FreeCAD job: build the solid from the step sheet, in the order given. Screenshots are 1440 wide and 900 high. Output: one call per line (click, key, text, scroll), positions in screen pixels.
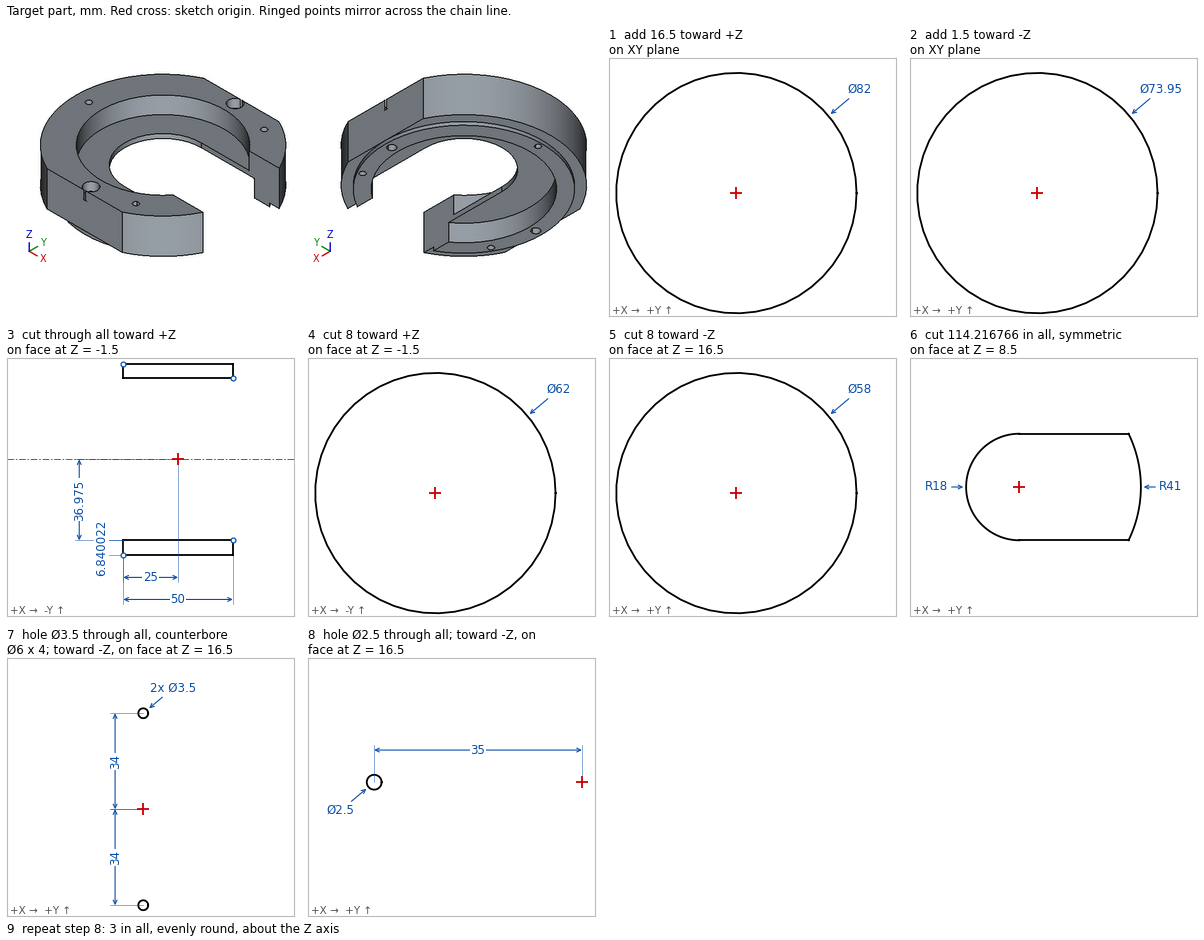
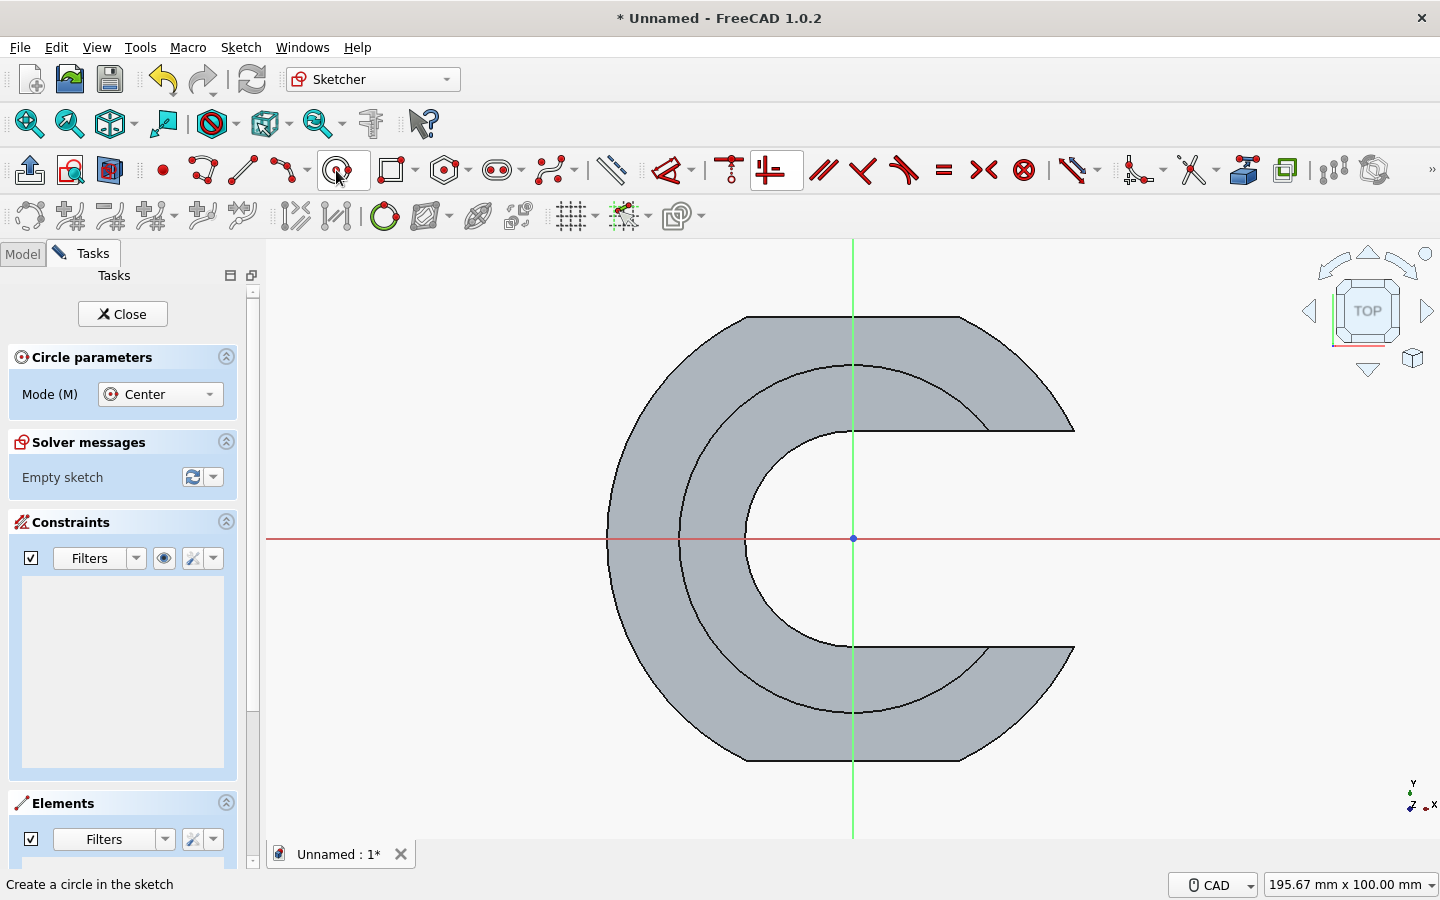
scroll(853, 335, up, 4)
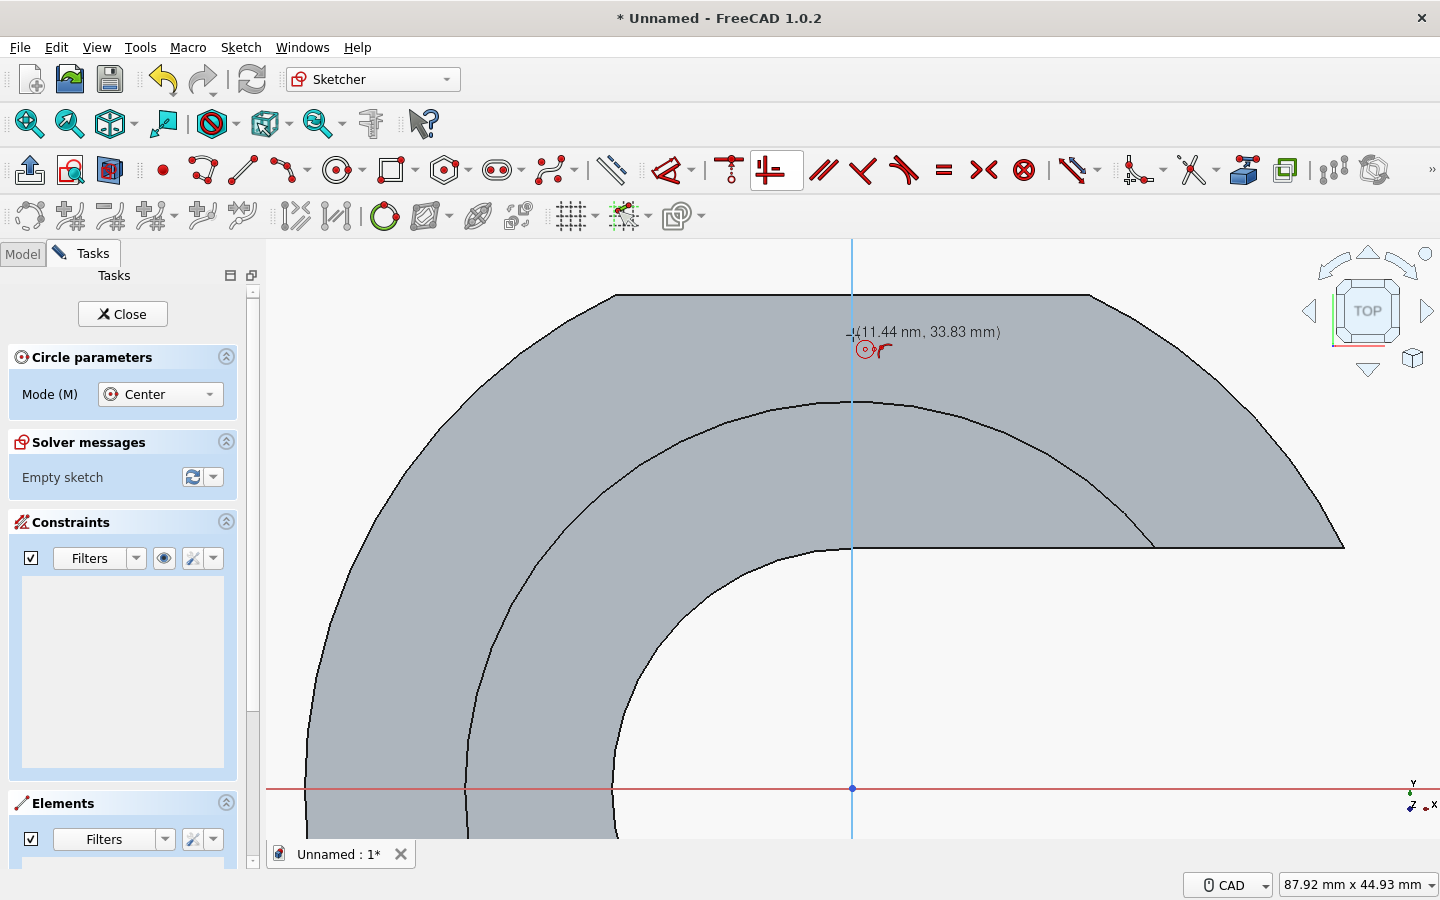
click(852, 335)
click(869, 318)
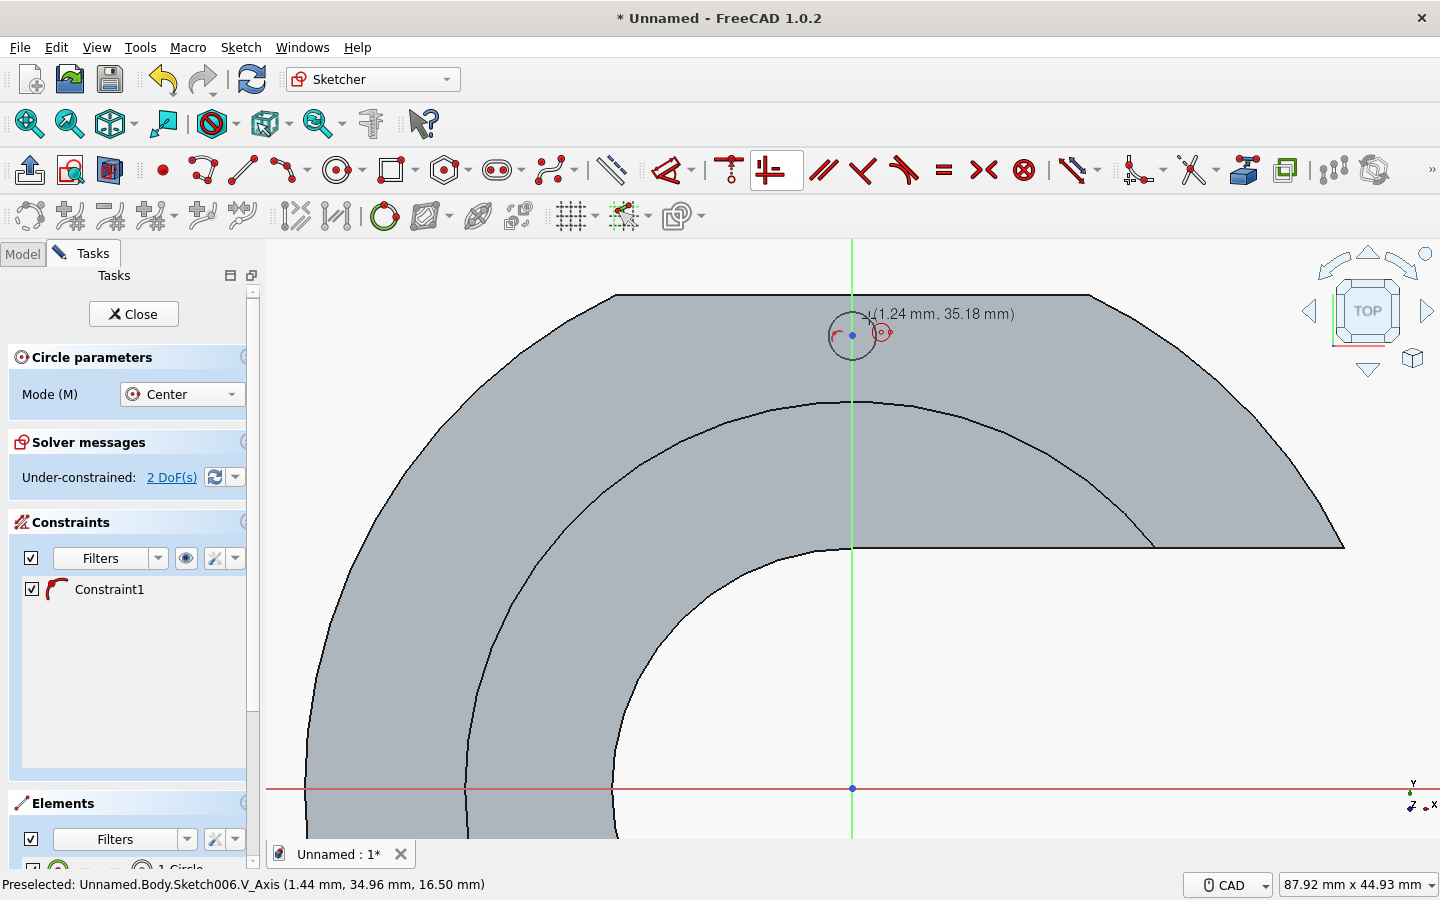
scroll(745, 394, down, 5)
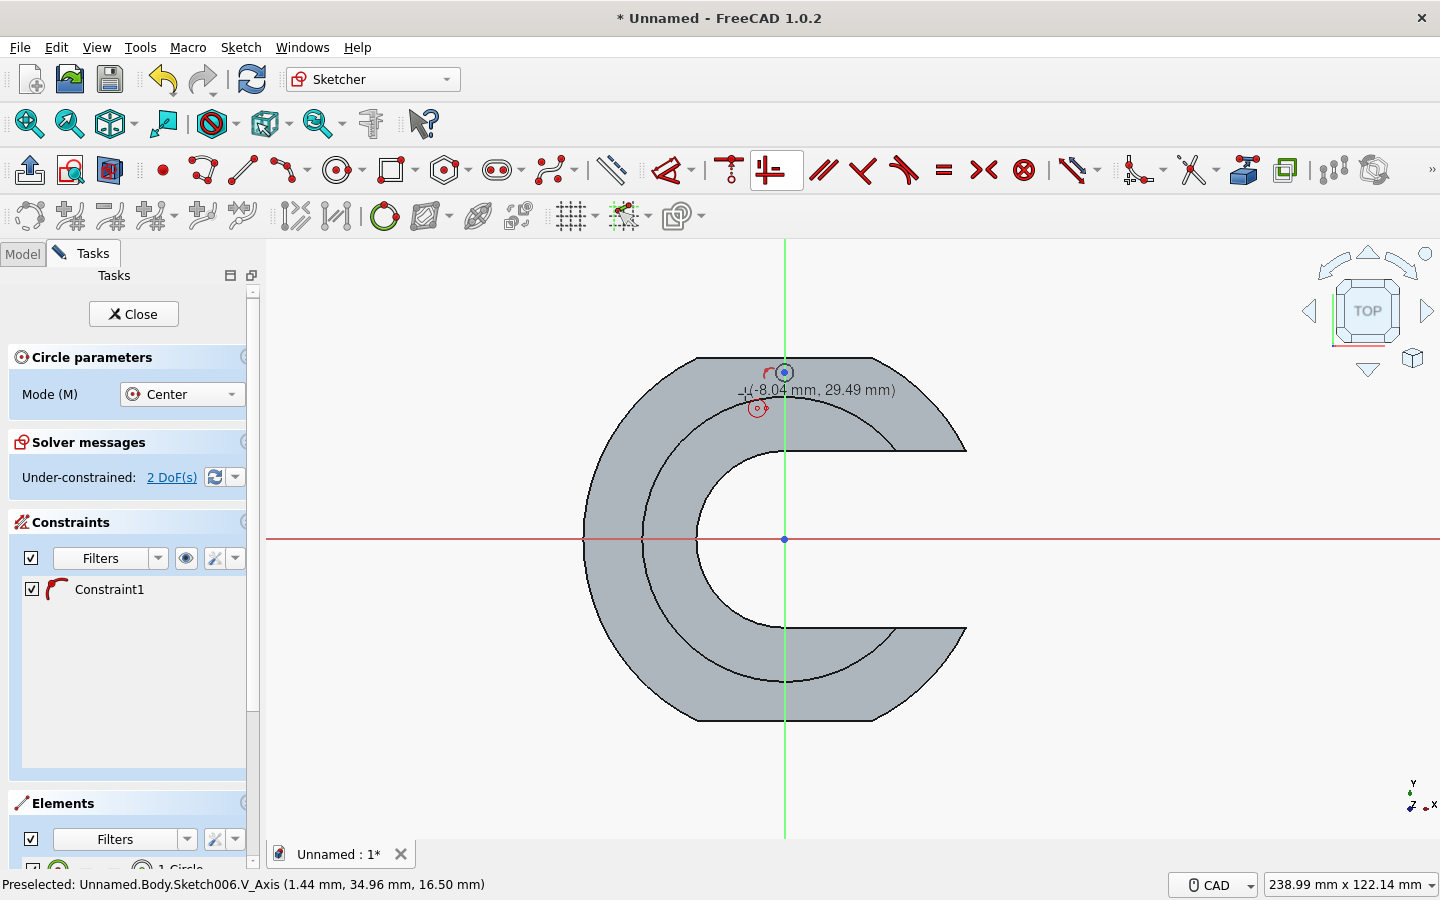
scroll(785, 706, up, 5)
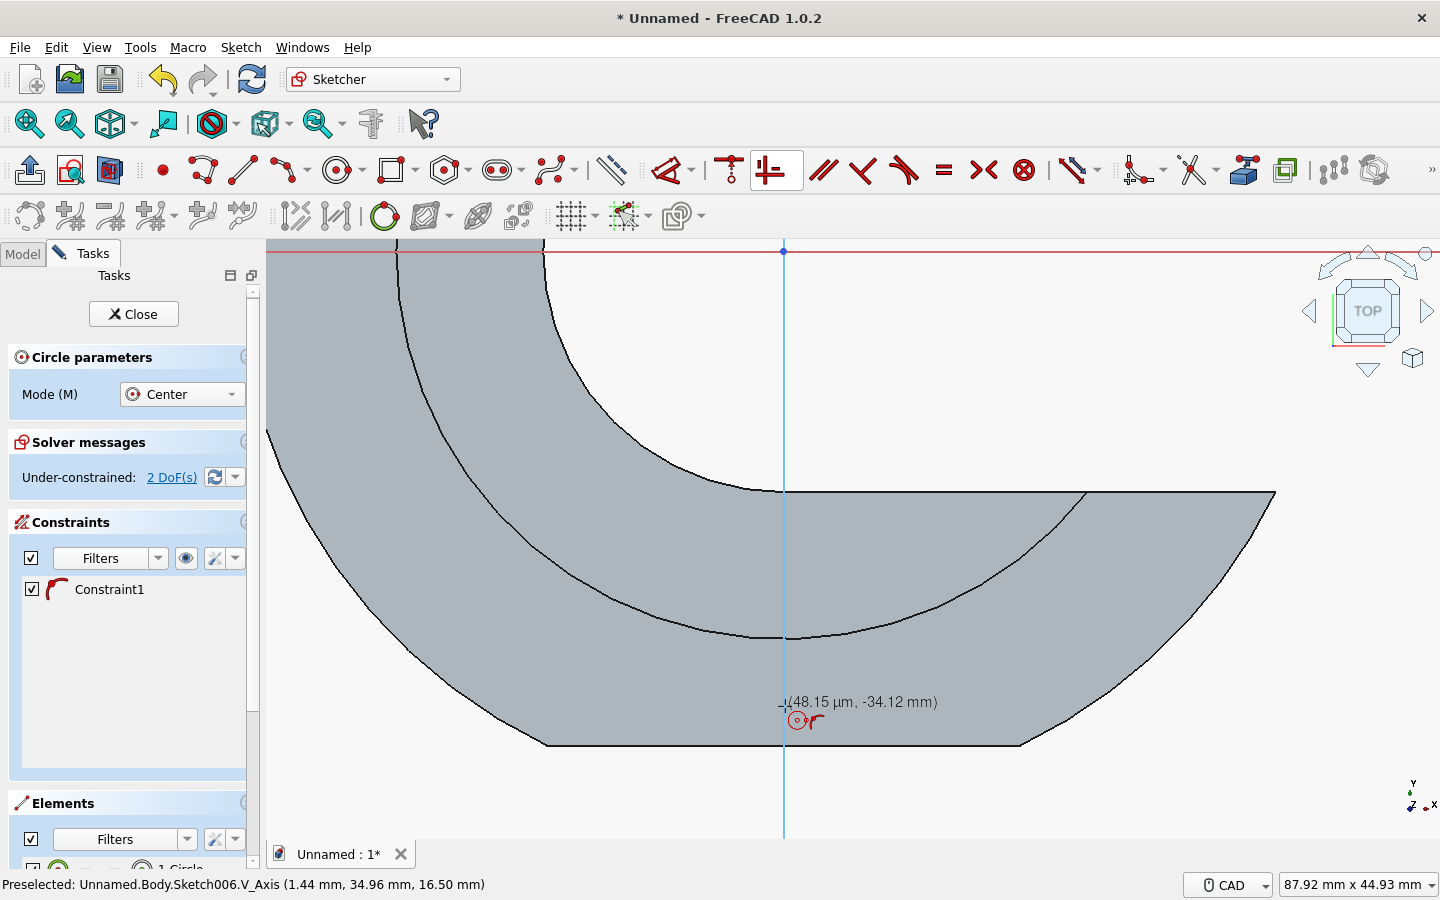
click(784, 706)
click(800, 689)
key(Escape)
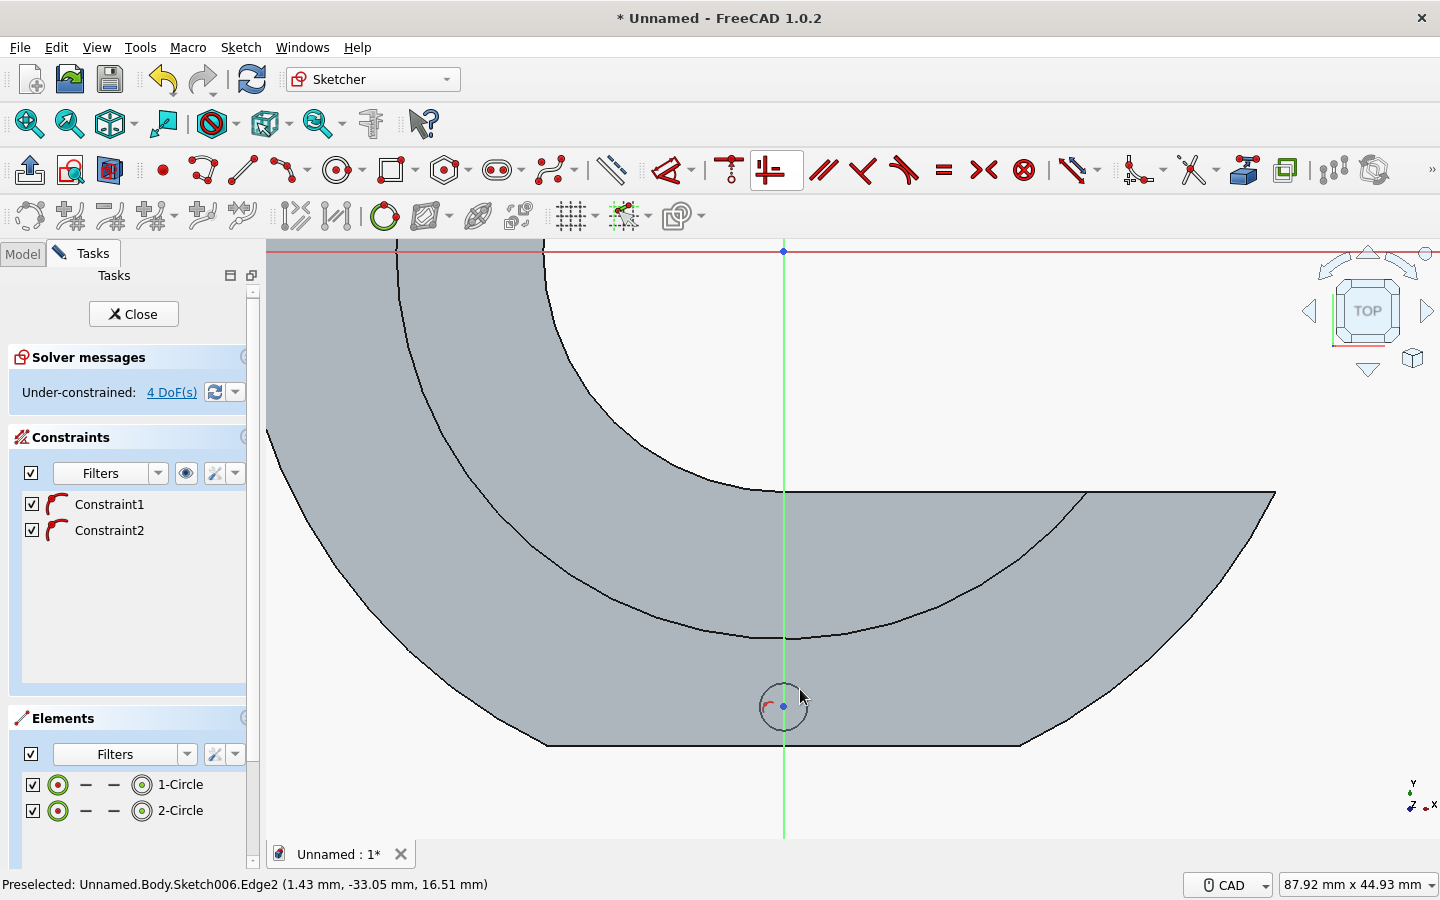
scroll(785, 706, down, 5)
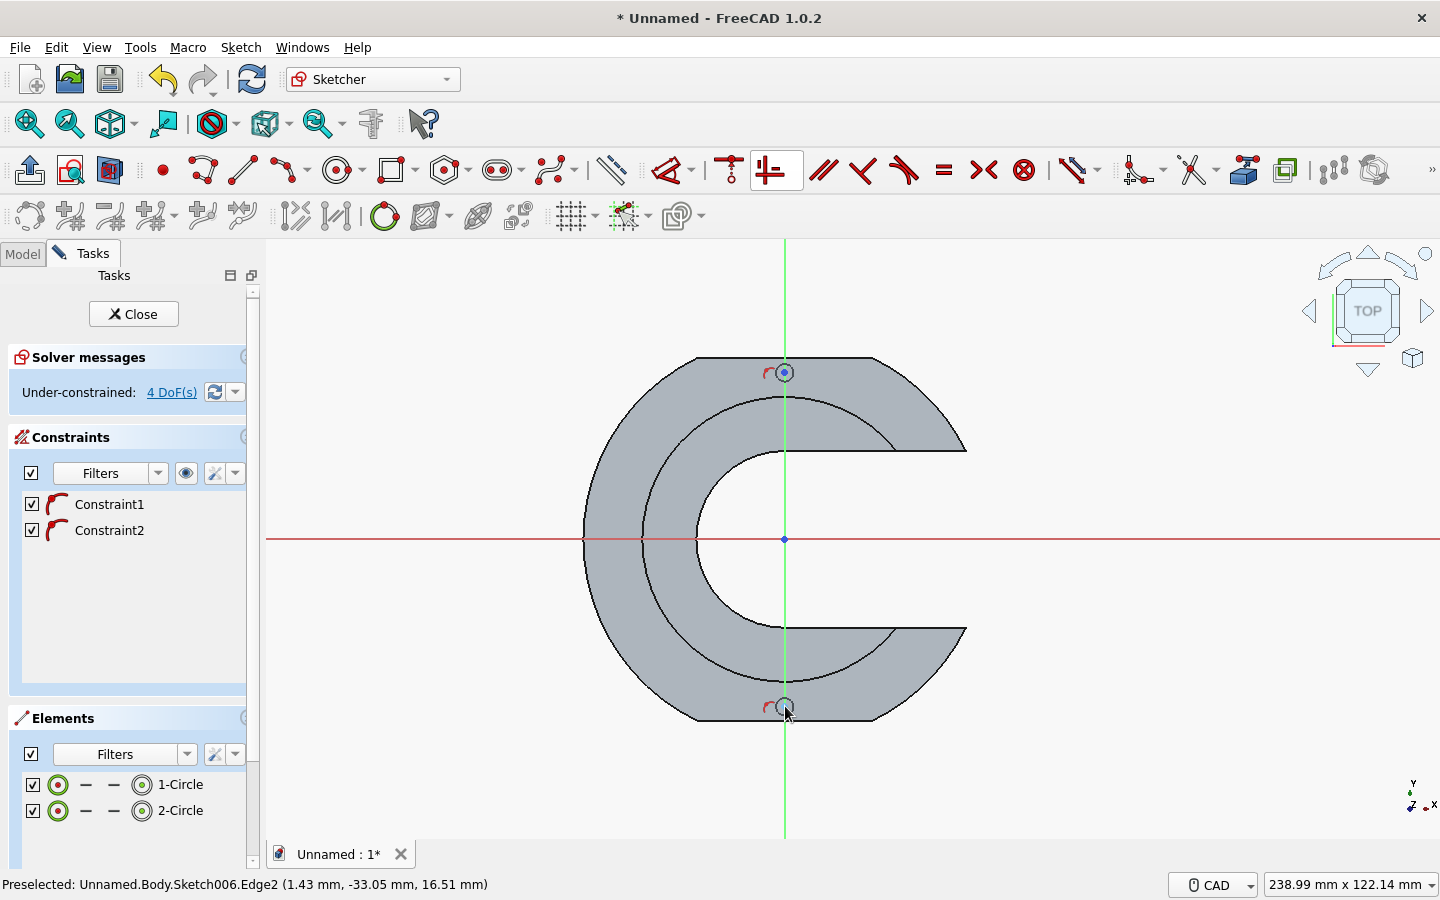
scroll(791, 367, up, 5)